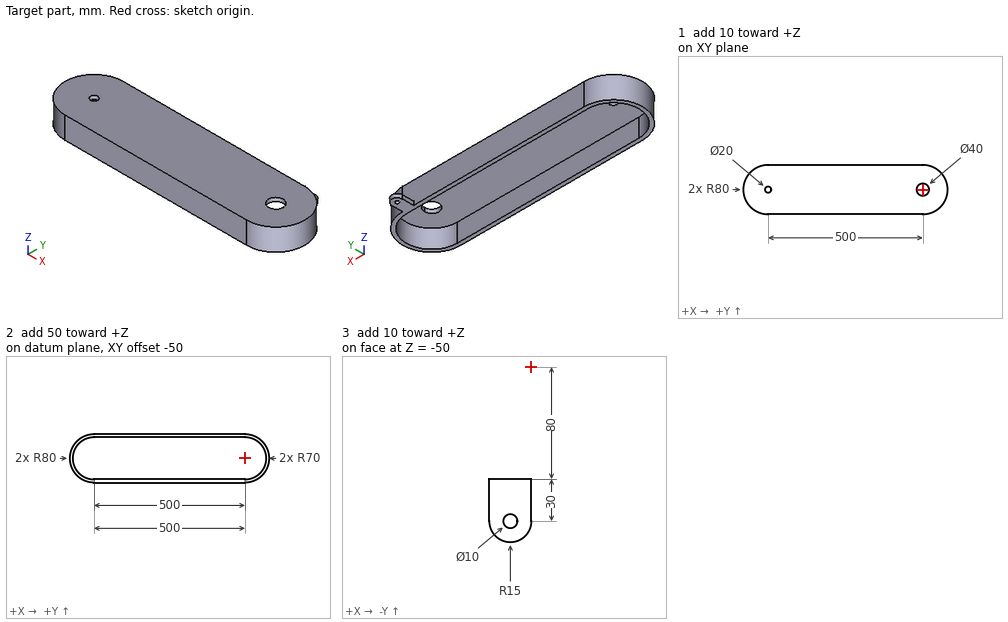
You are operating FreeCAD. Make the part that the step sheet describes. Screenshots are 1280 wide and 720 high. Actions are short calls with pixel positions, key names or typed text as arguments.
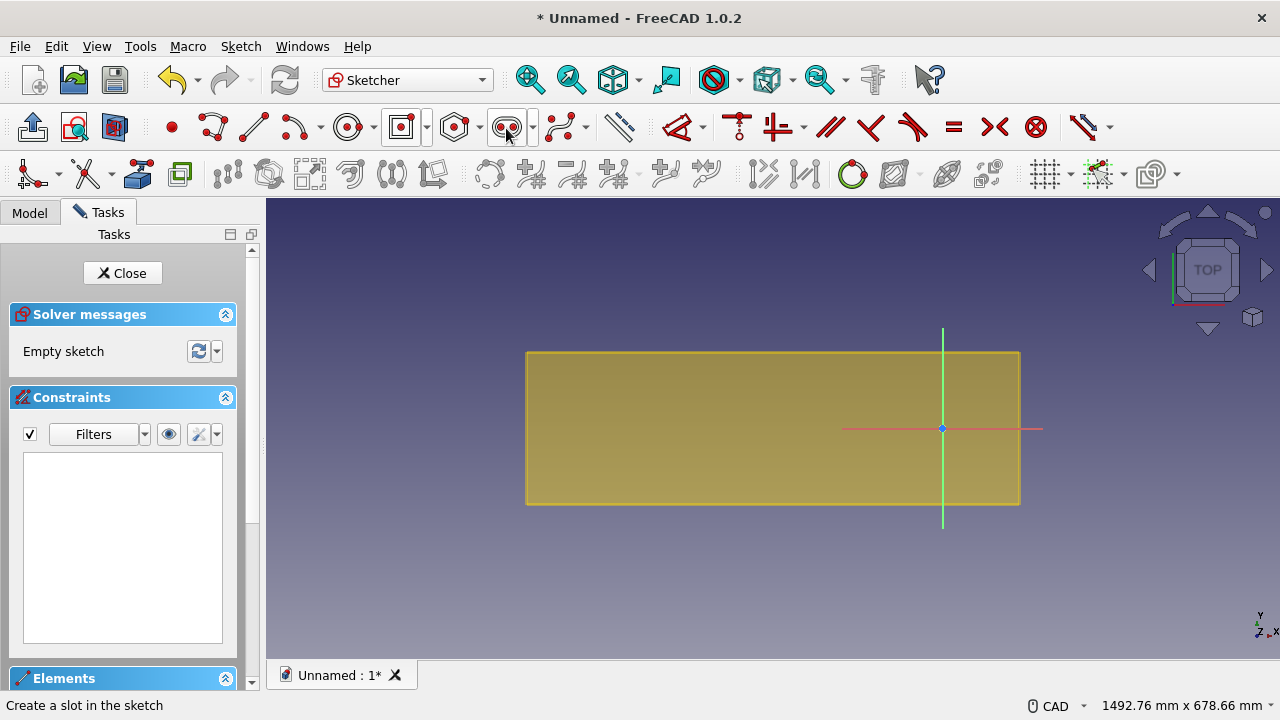
click(943, 428)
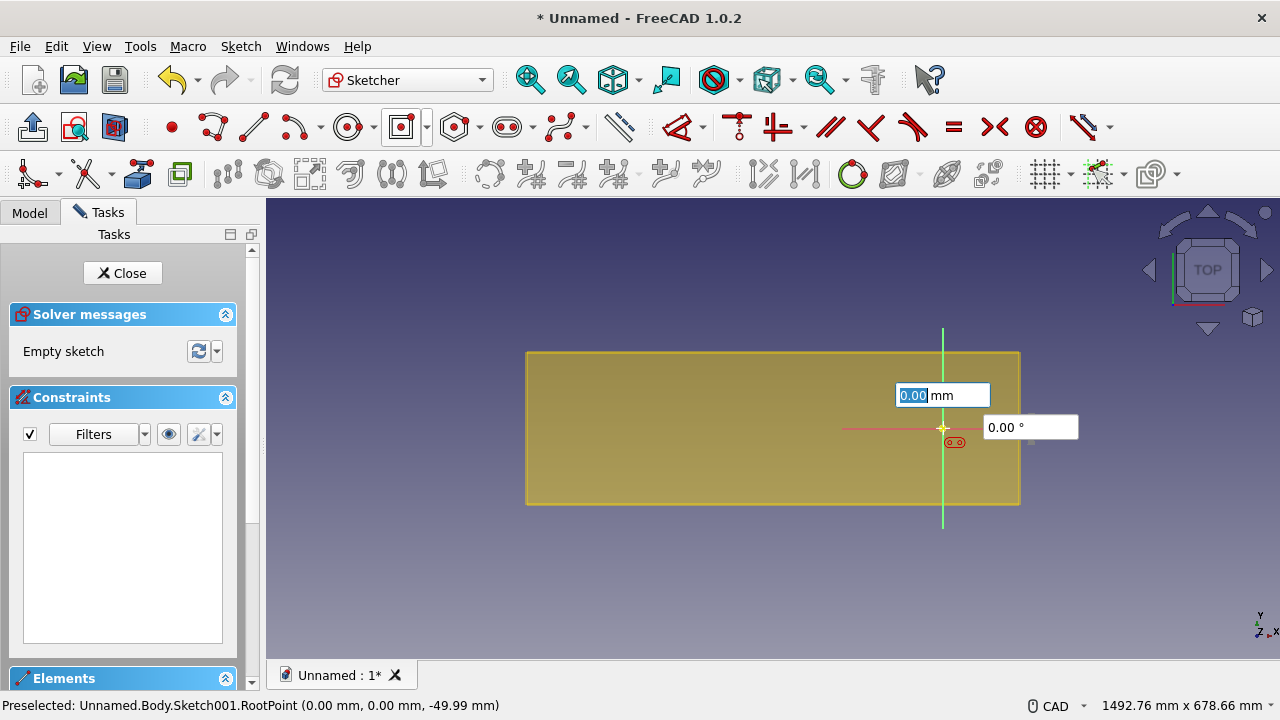
click(603, 420)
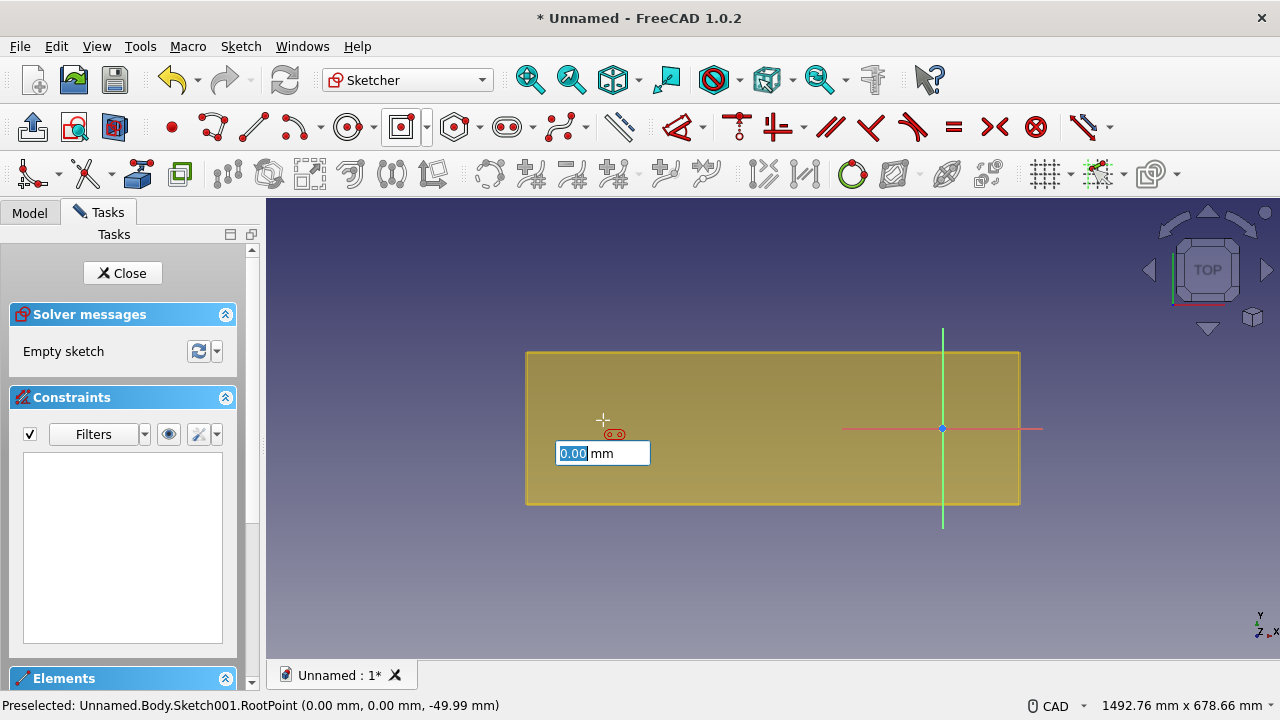
click(773, 483)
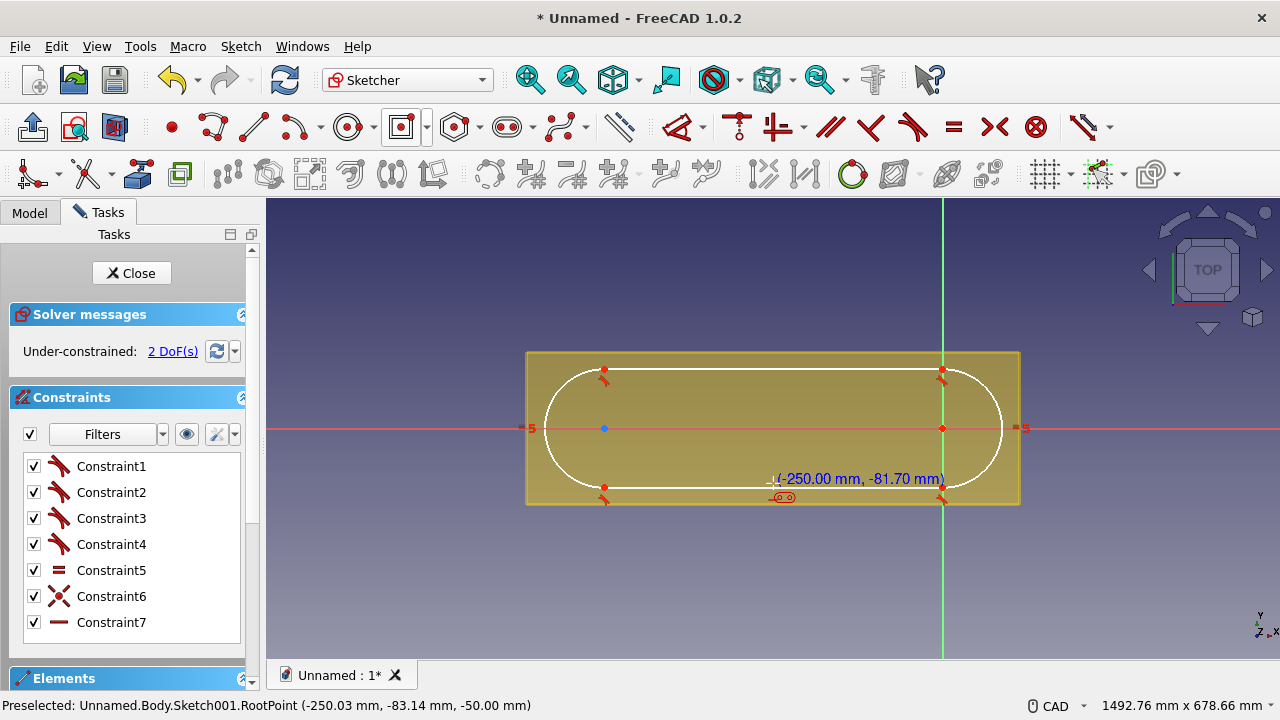
click(943, 428)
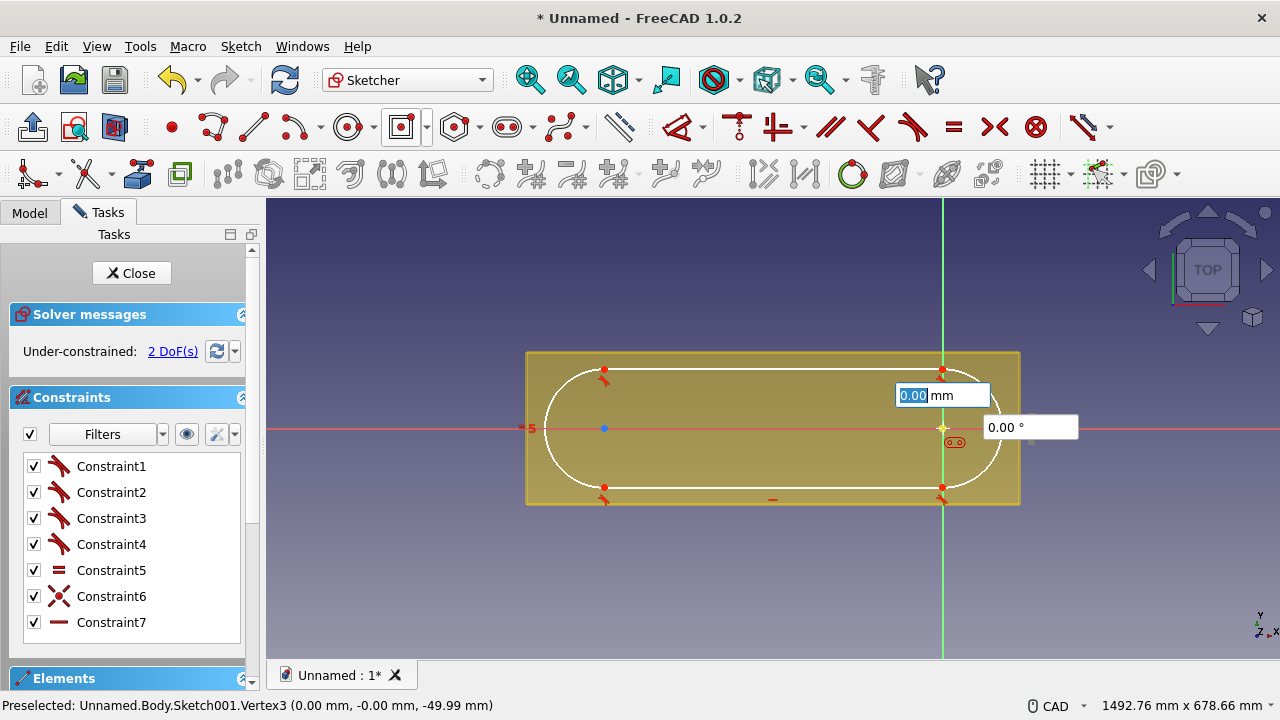
click(604, 428)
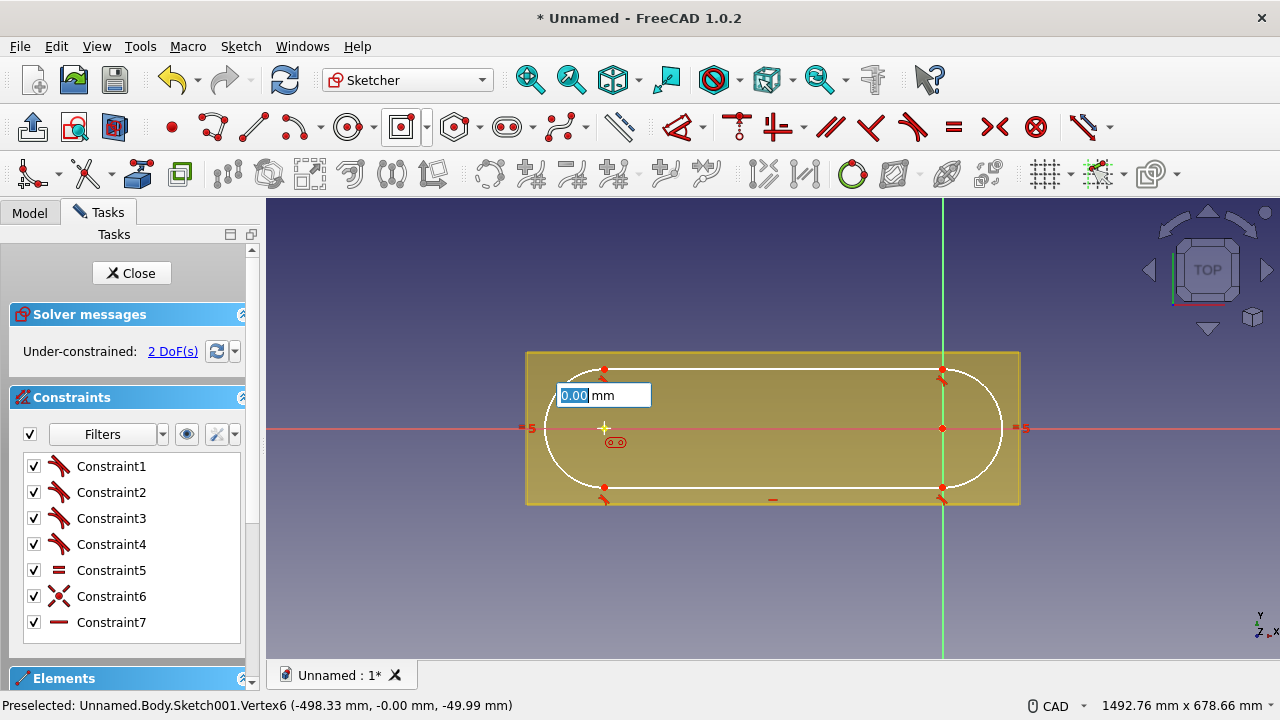
scroll(773, 476, up, 5)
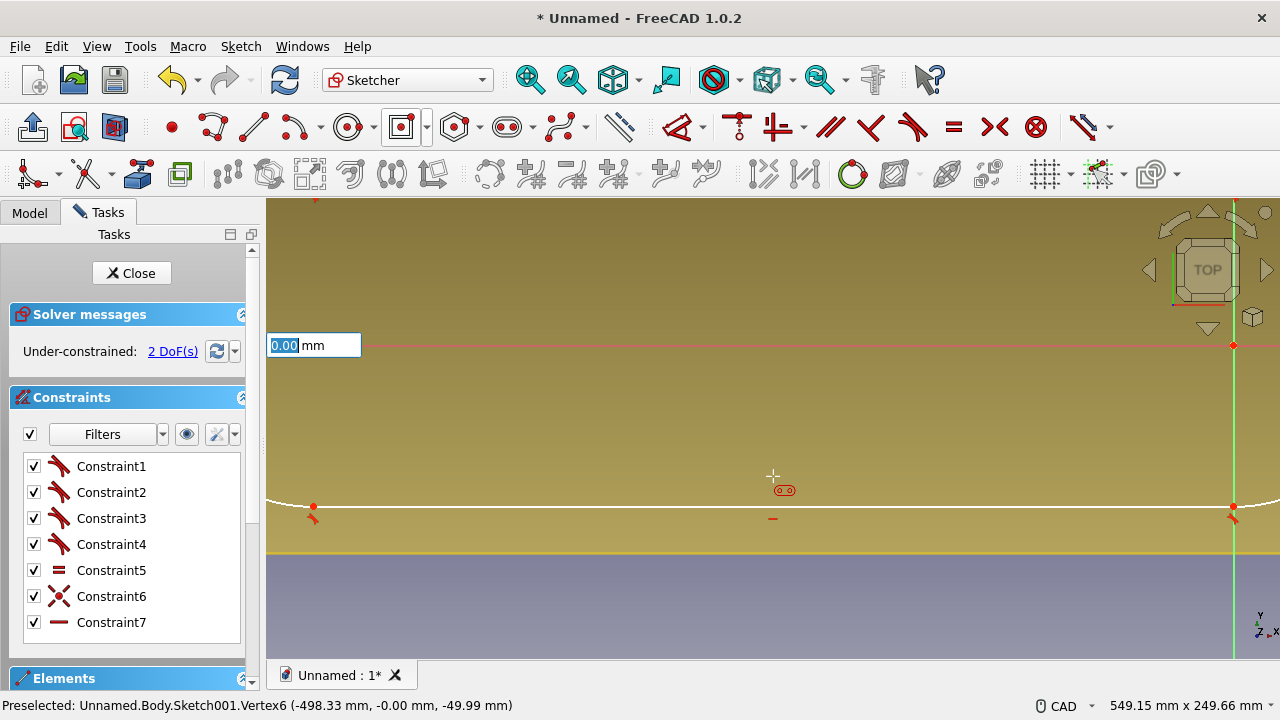
click(772, 475)
key(Escape)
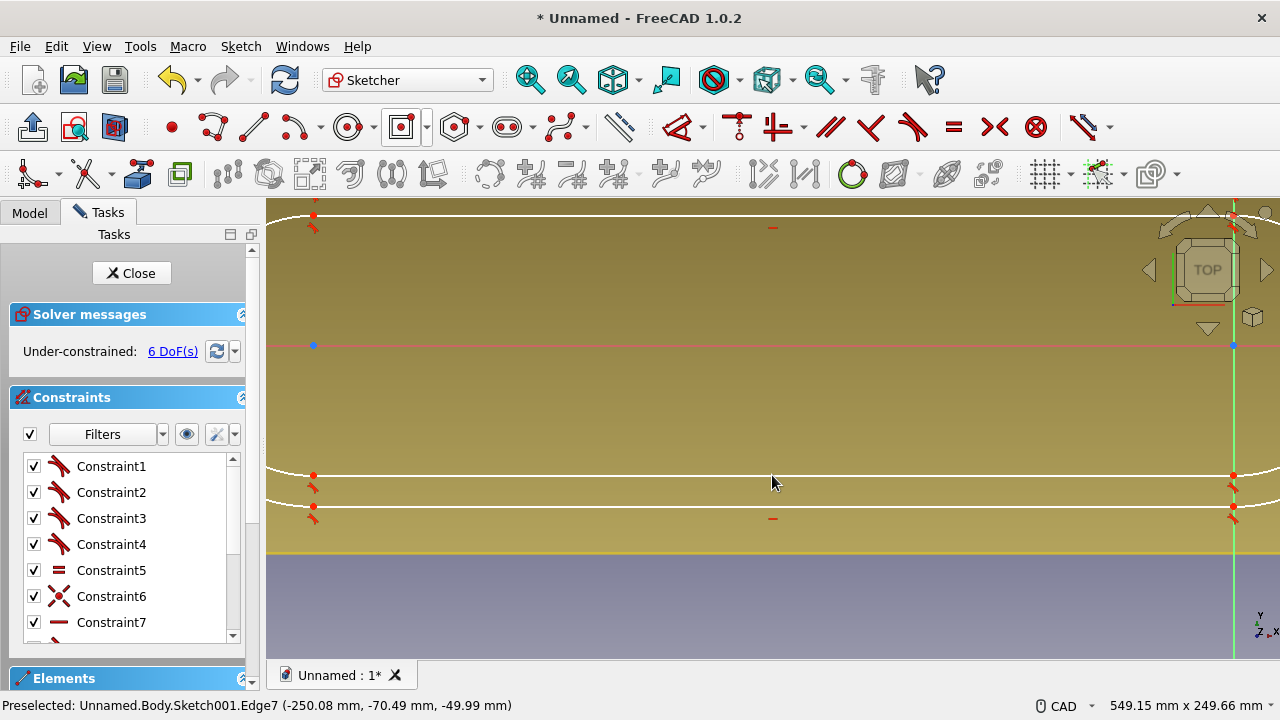
scroll(649, 496, down, 4)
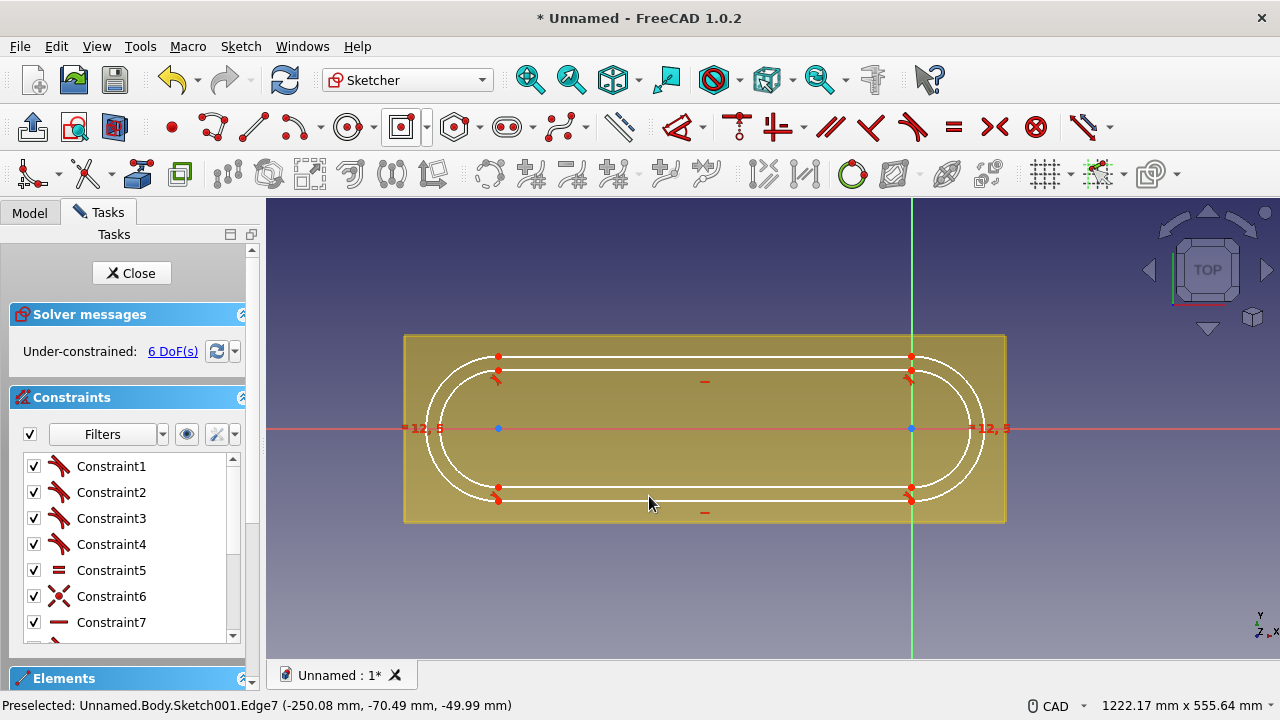
click(971, 471)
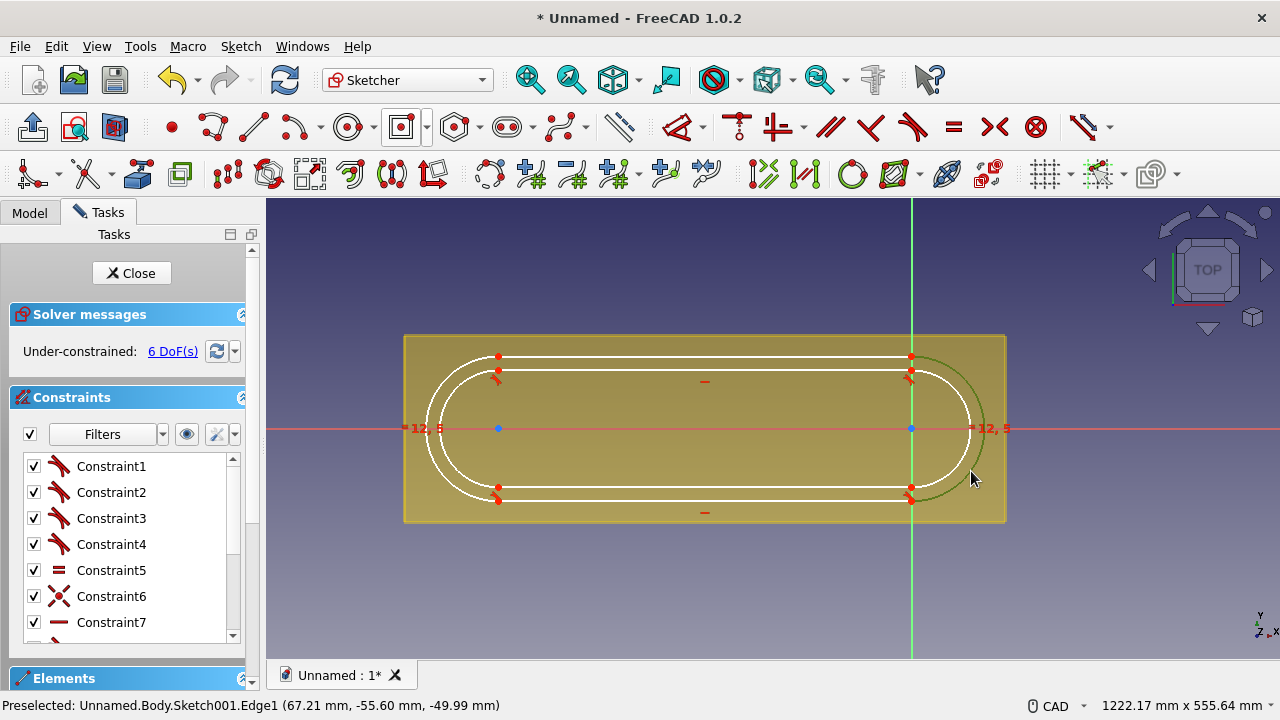
click(959, 463)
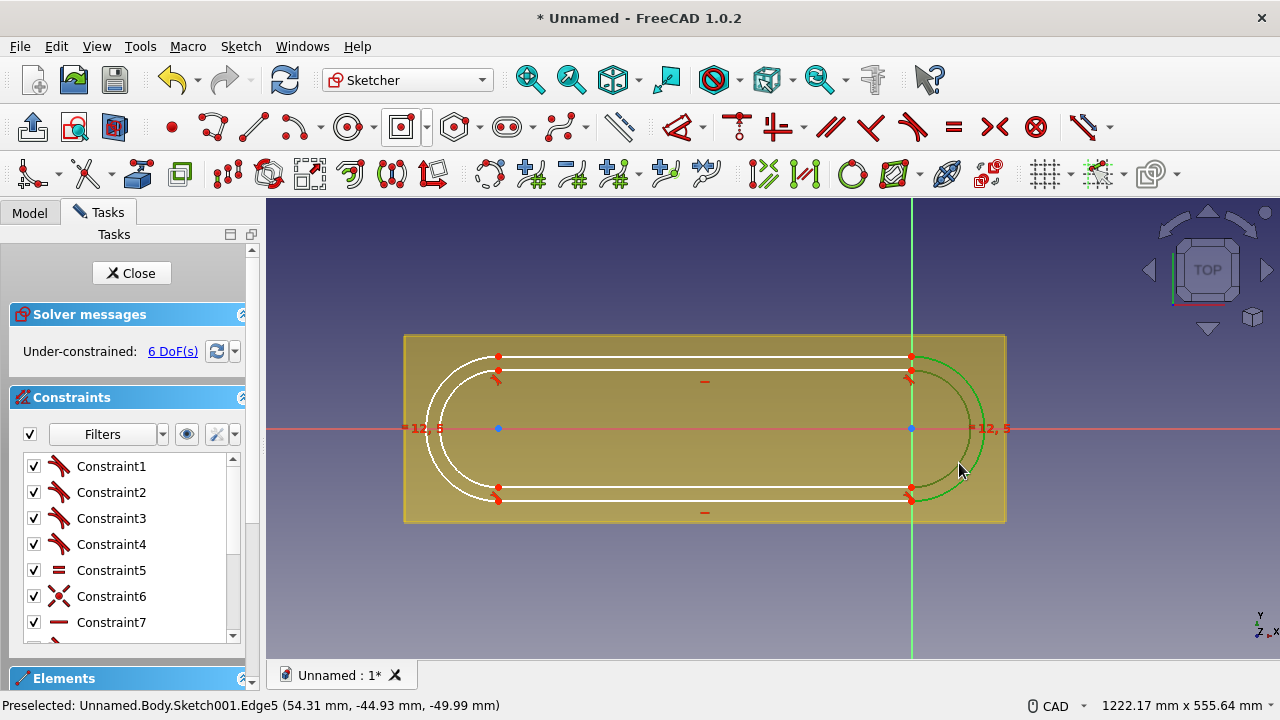
key(c)